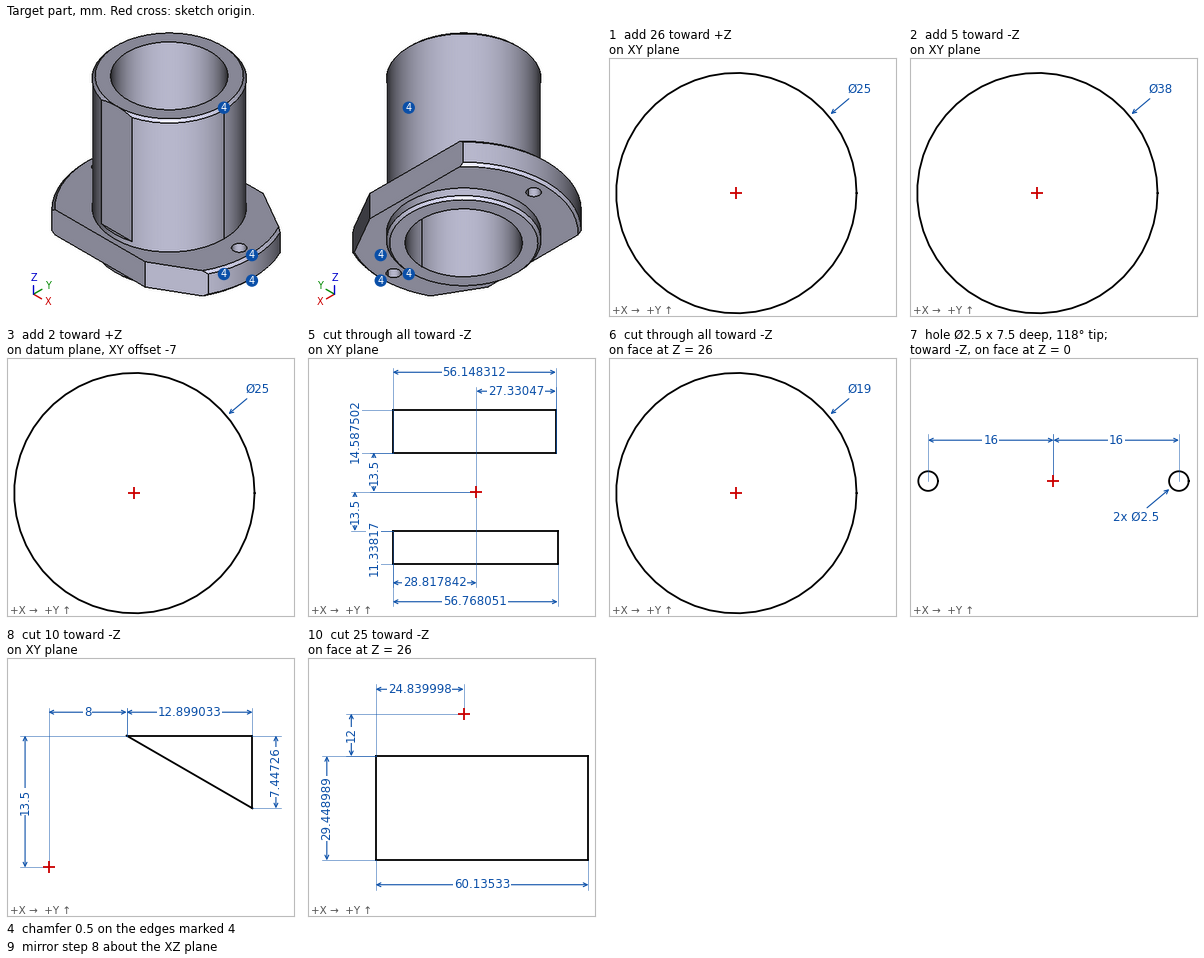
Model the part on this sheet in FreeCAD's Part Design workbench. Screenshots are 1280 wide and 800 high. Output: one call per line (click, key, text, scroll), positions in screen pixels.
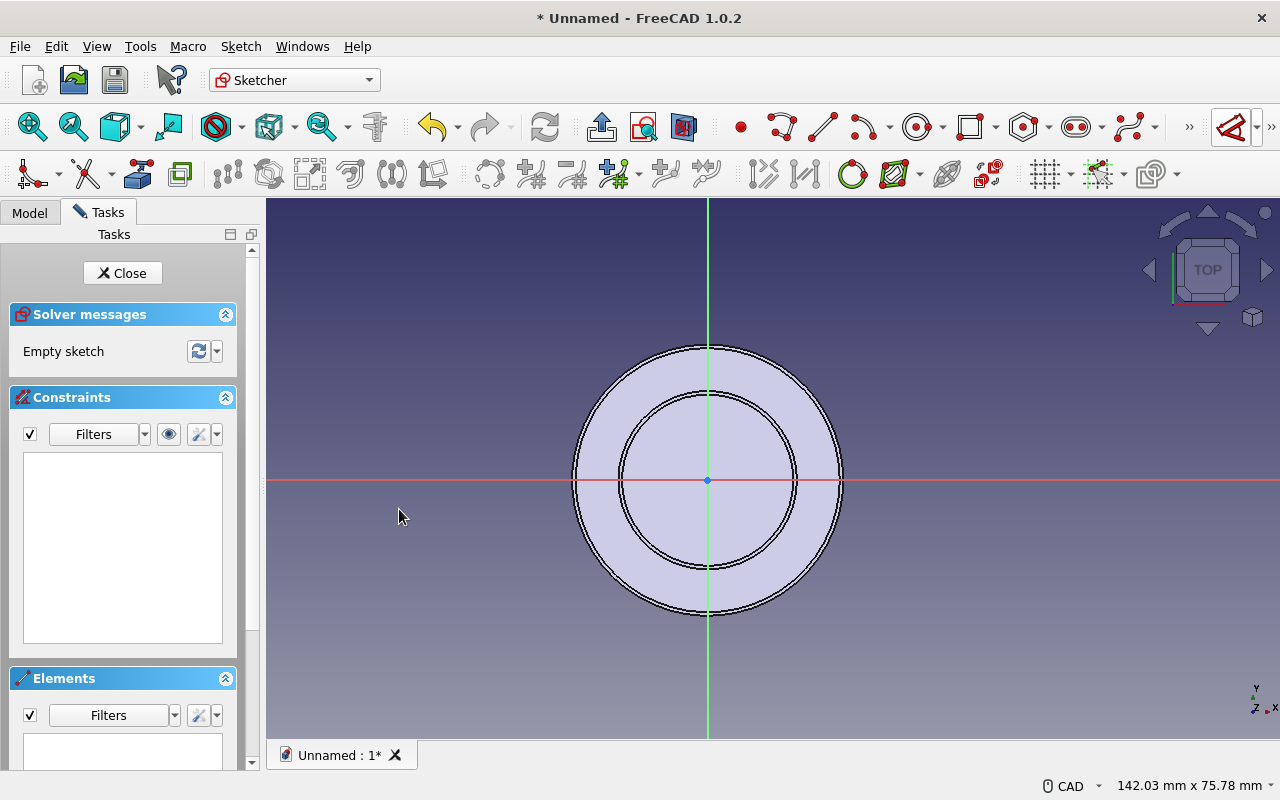
click(970, 128)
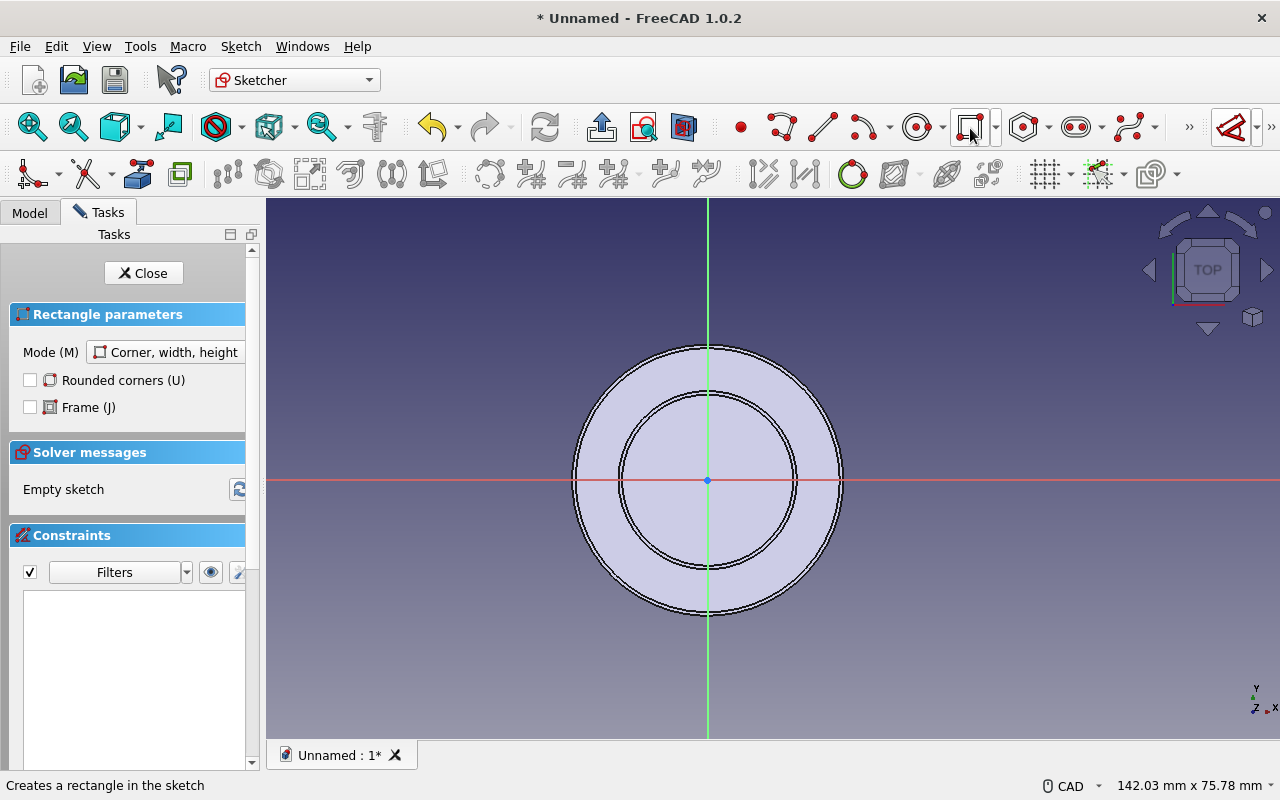
click(502, 577)
click(907, 658)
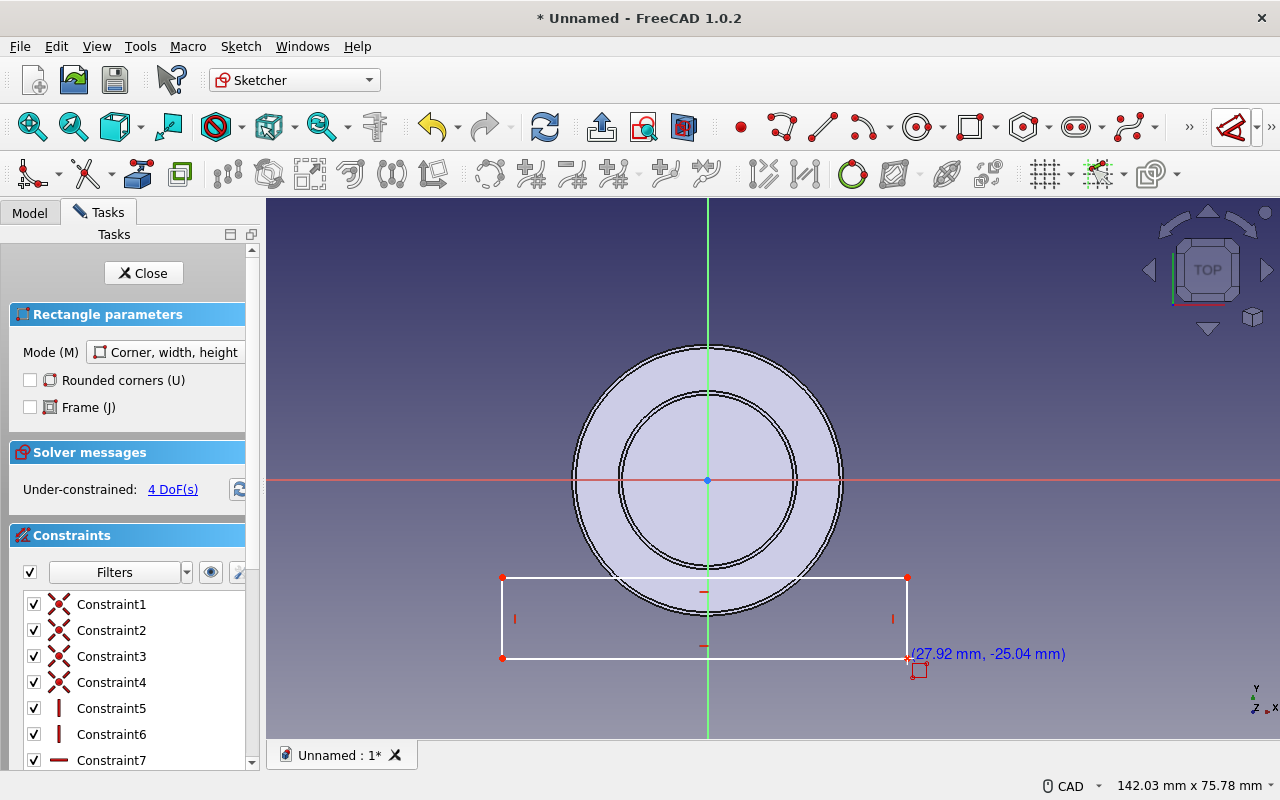
click(502, 280)
click(903, 384)
key(Escape)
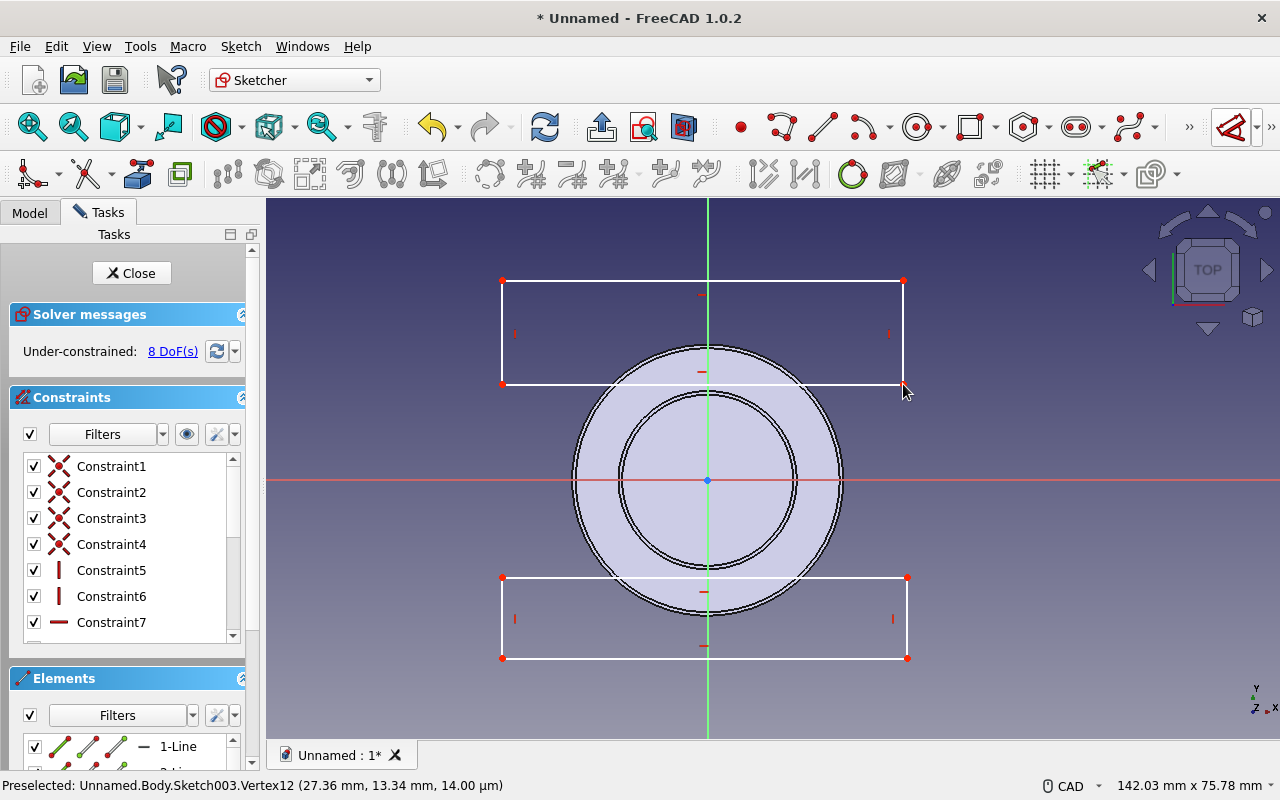
click(502, 578)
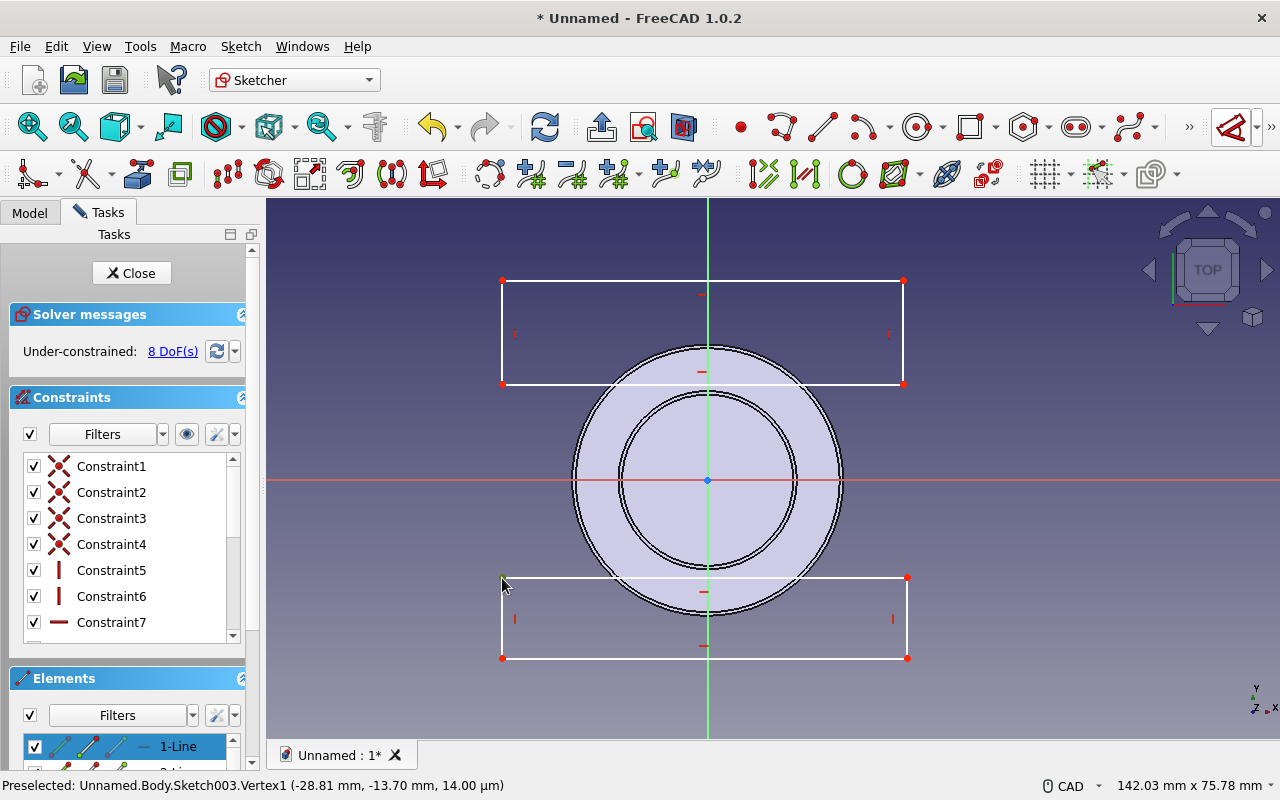
click(1256, 128)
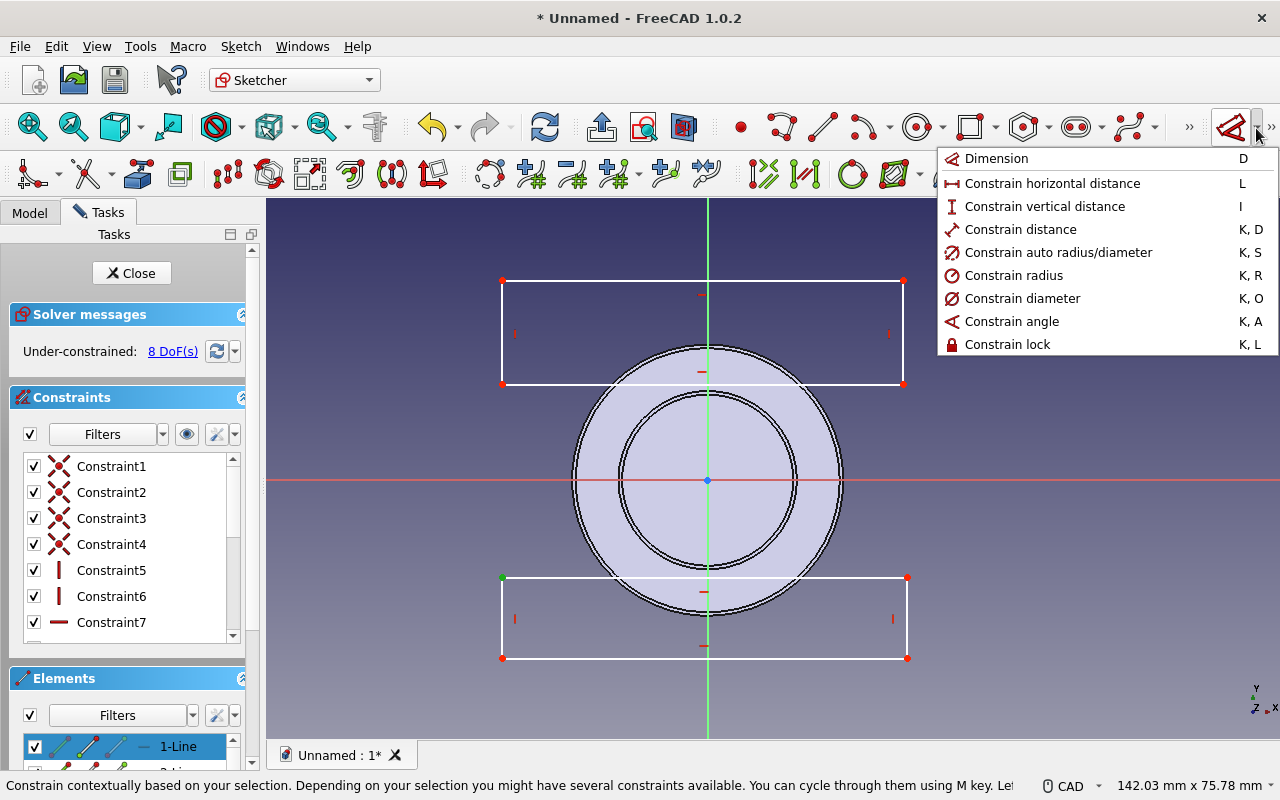
click(1108, 206)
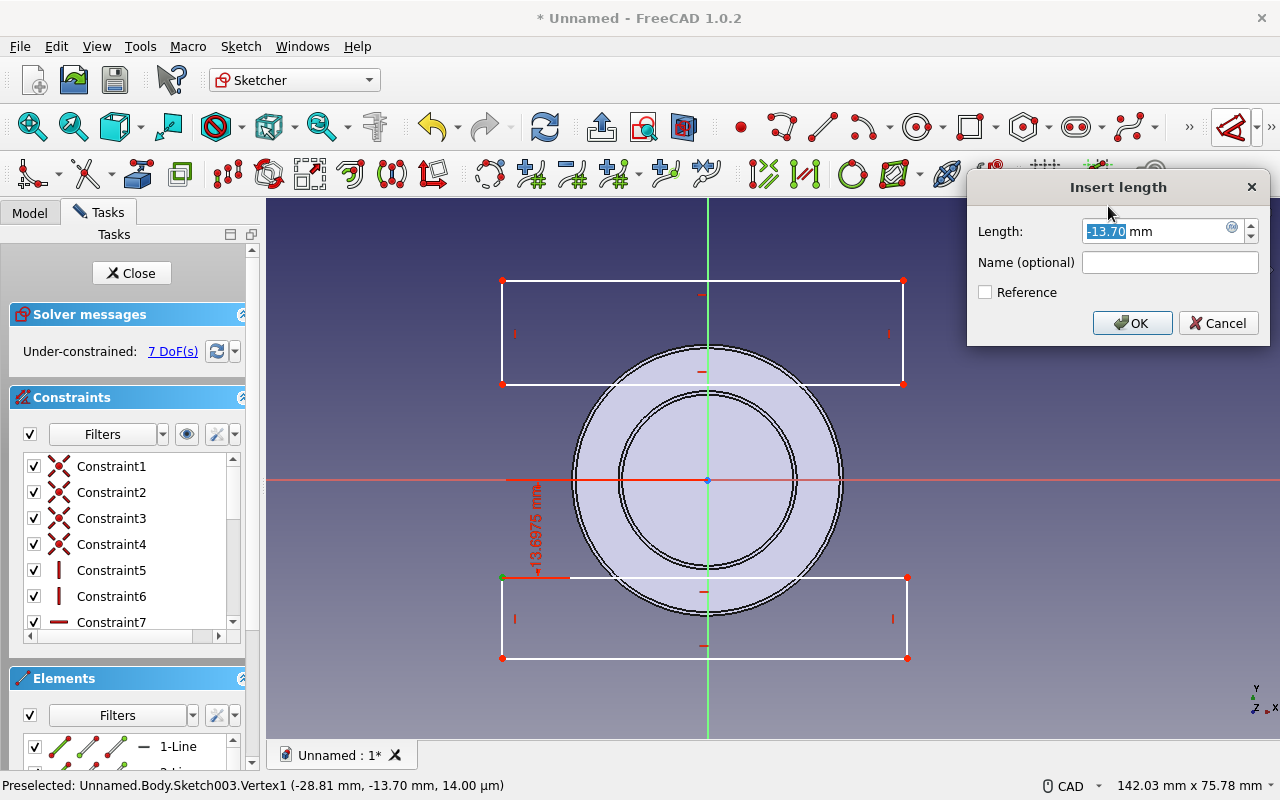
text(-13.5)
key(Return)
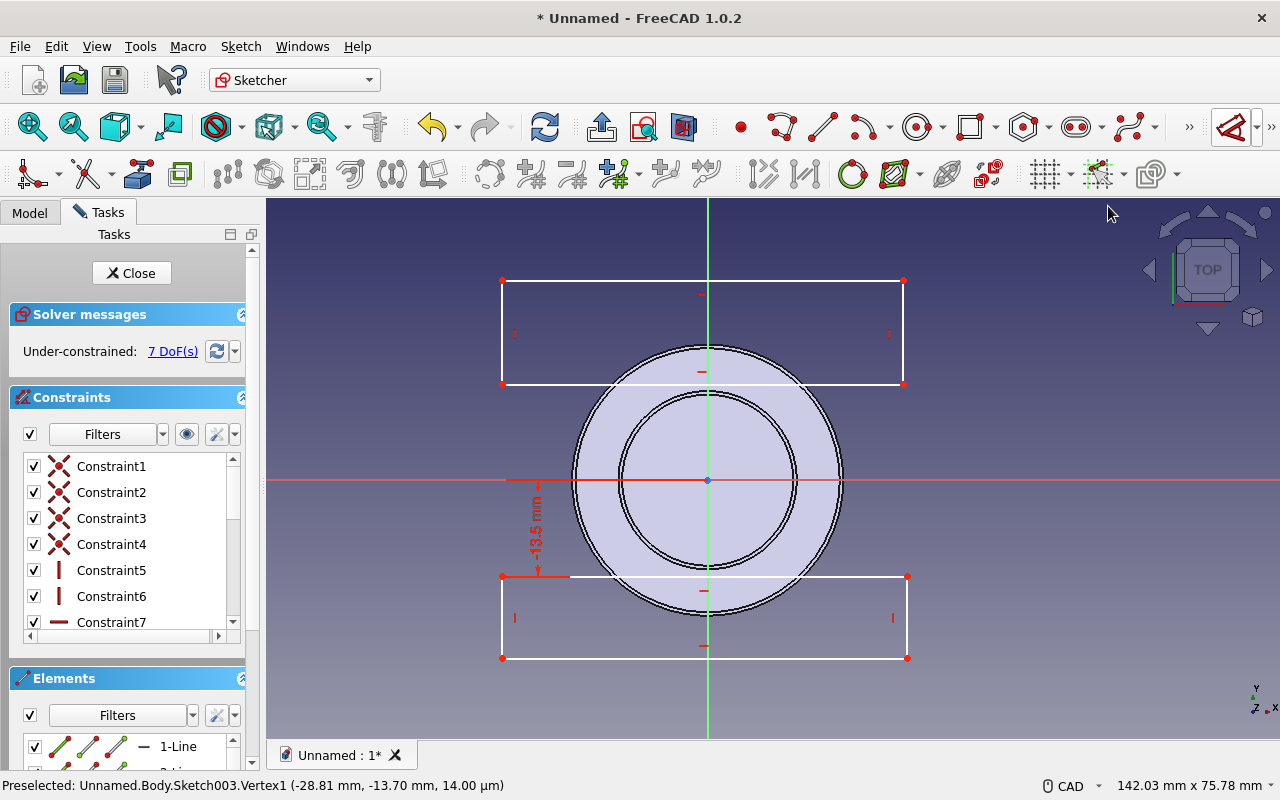
click(502, 385)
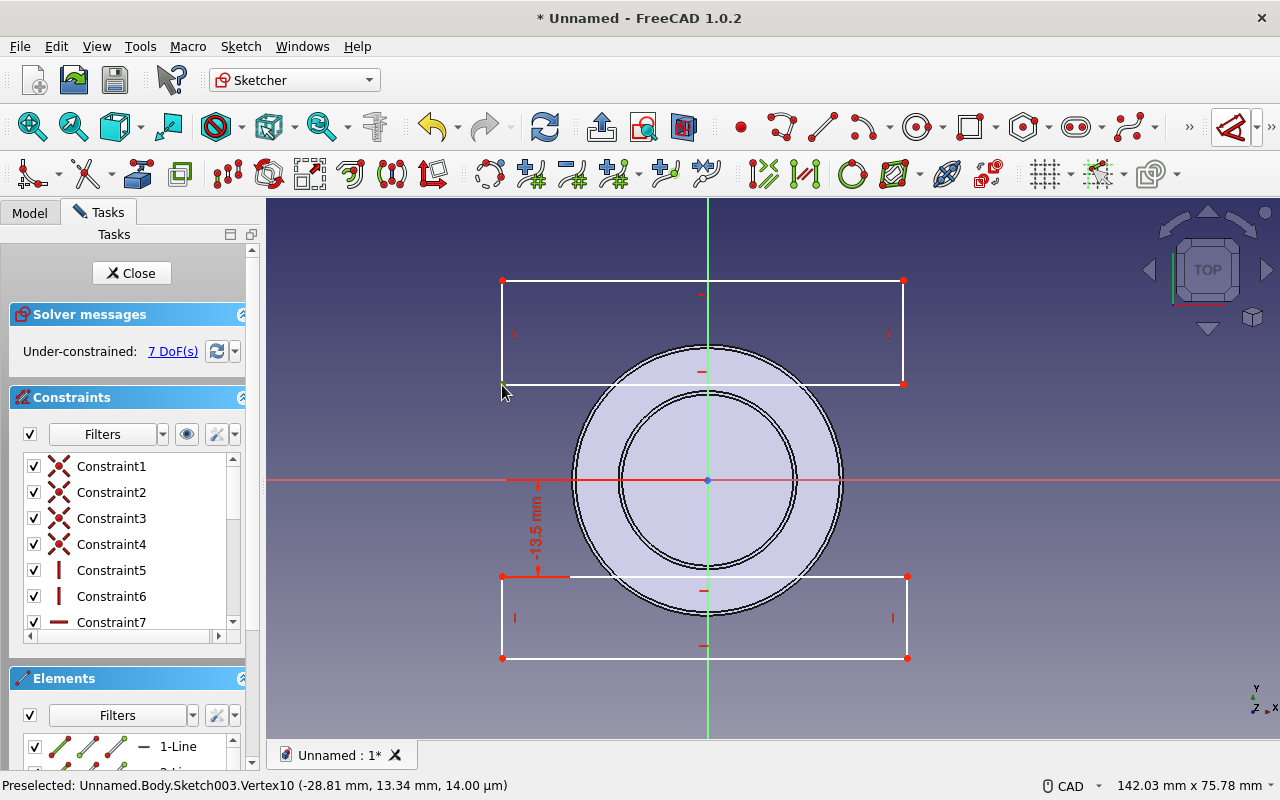
key(i)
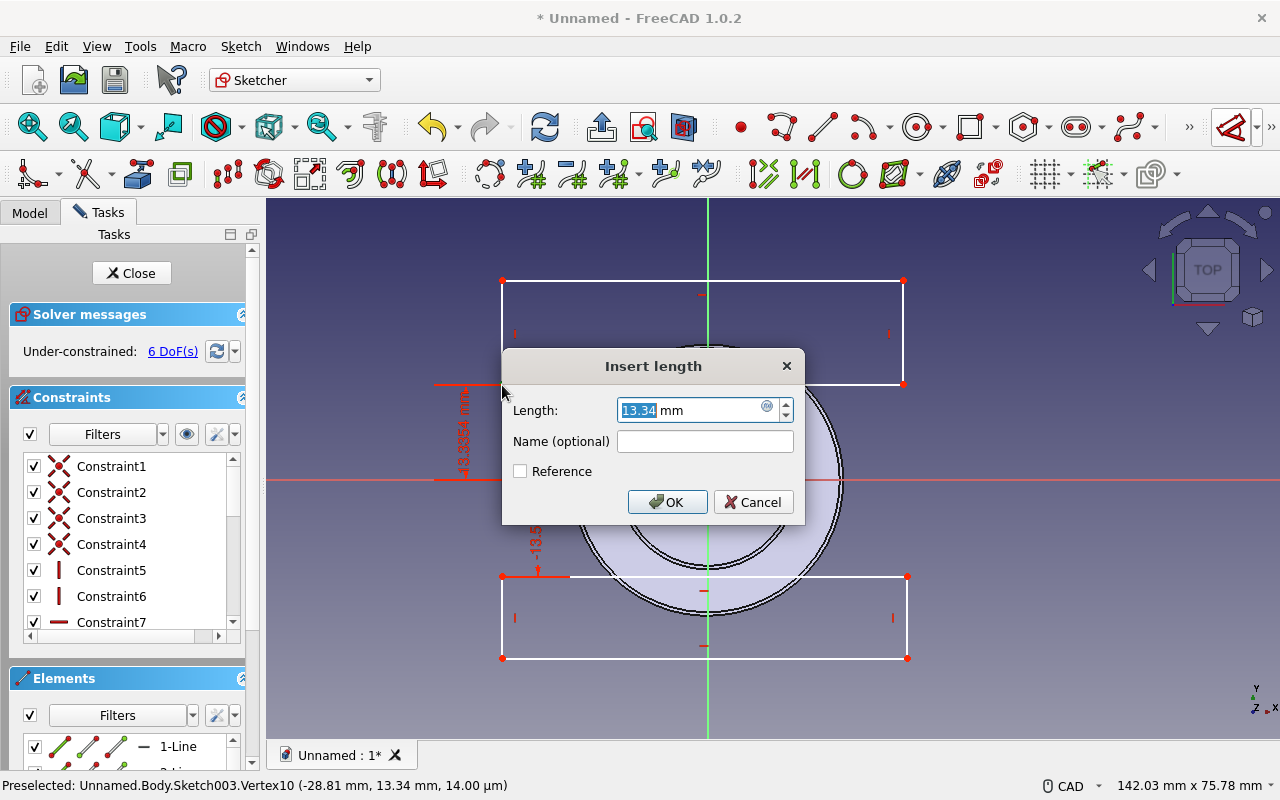
text(13.5)
key(Return)